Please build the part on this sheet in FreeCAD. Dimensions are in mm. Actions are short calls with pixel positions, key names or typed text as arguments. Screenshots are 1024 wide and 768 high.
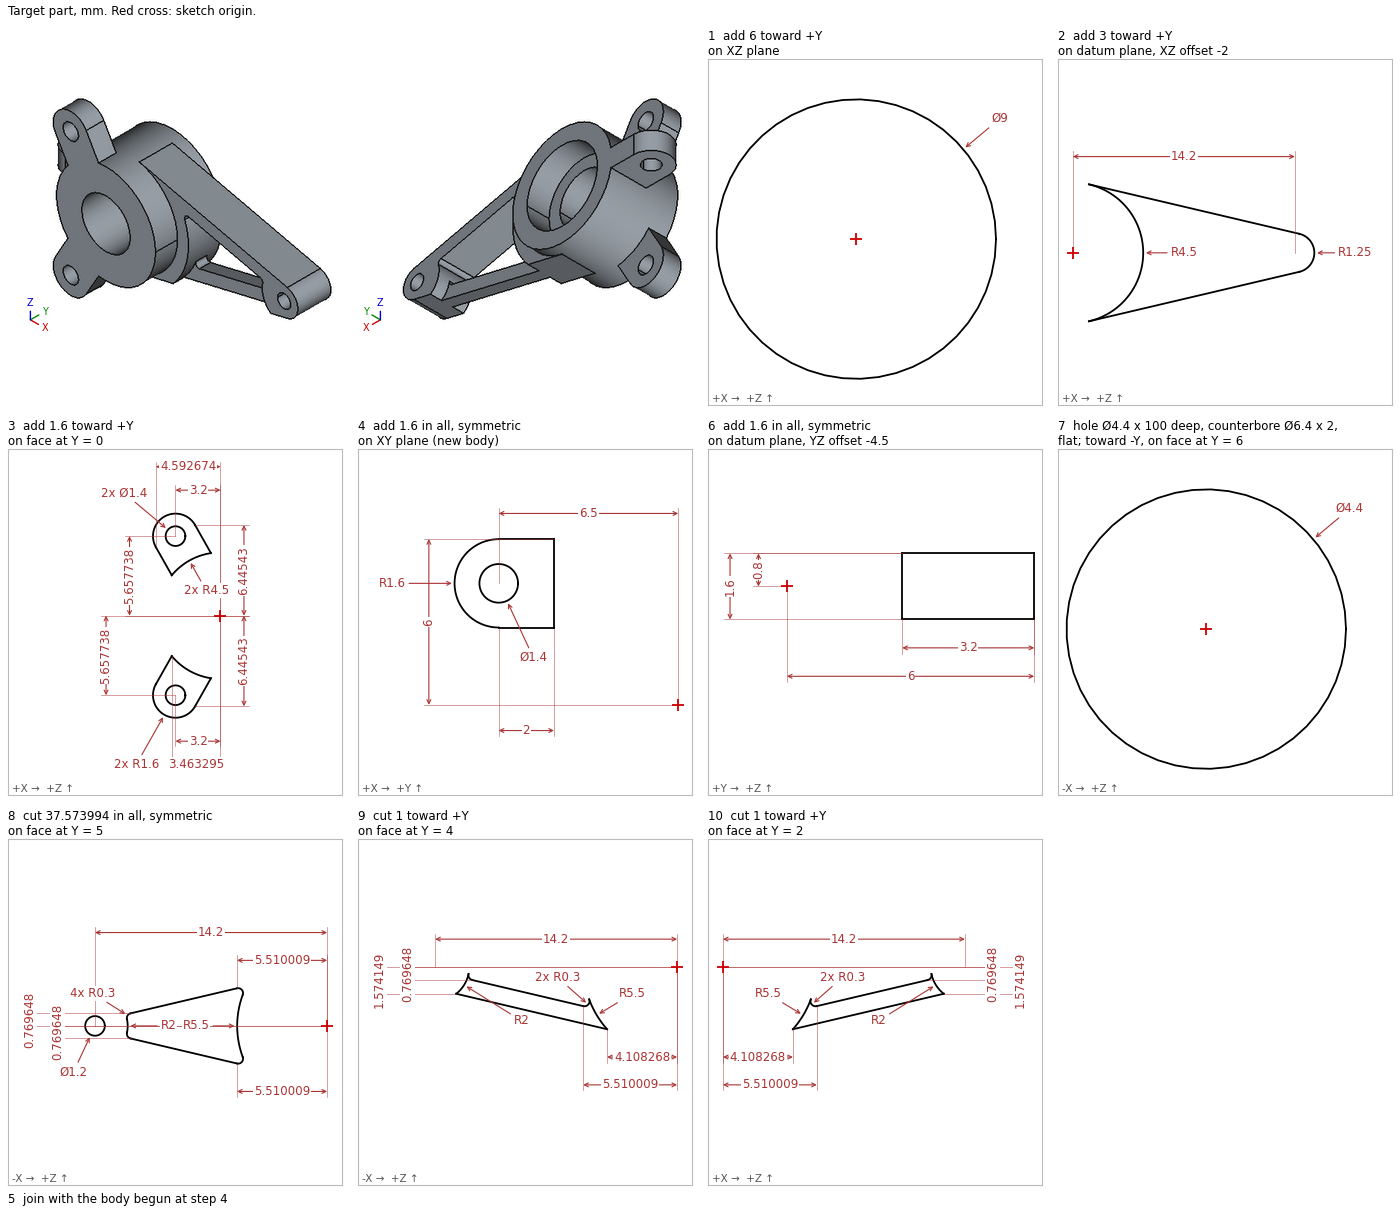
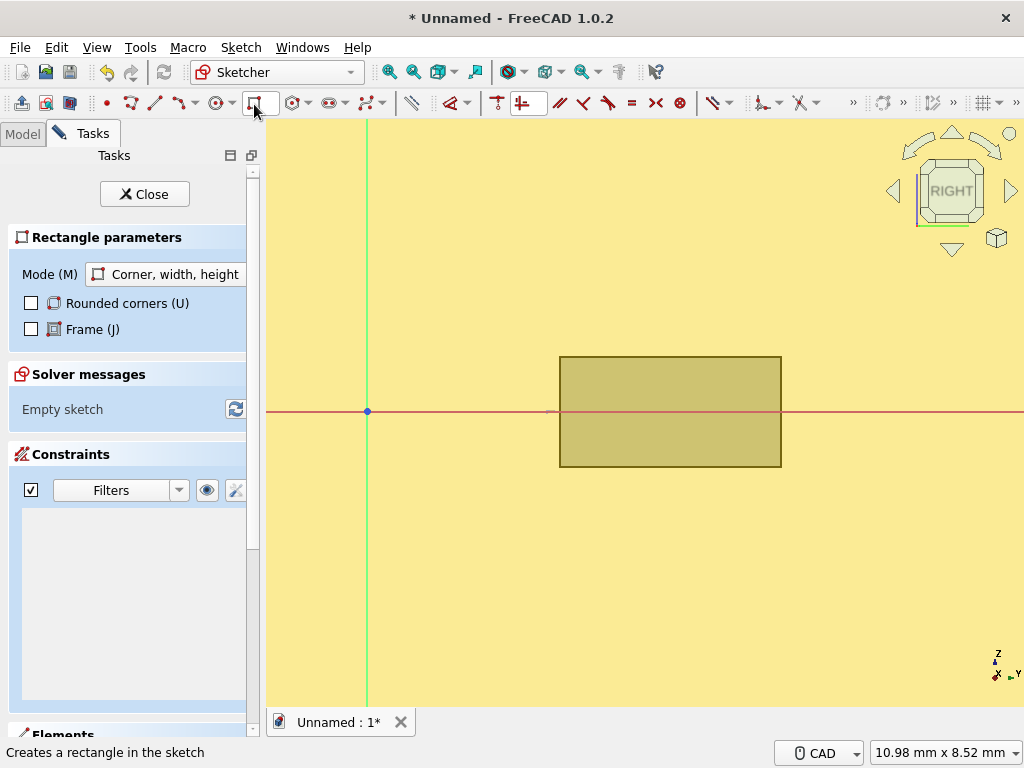
click(560, 357)
click(781, 467)
key(Escape)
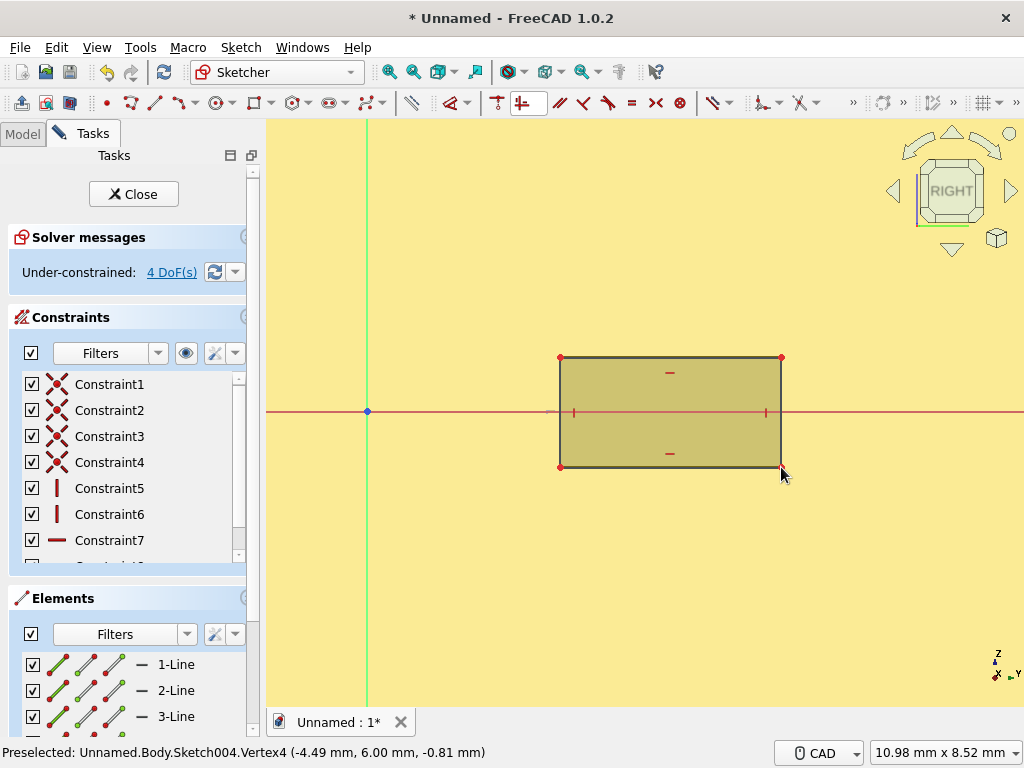
key(d)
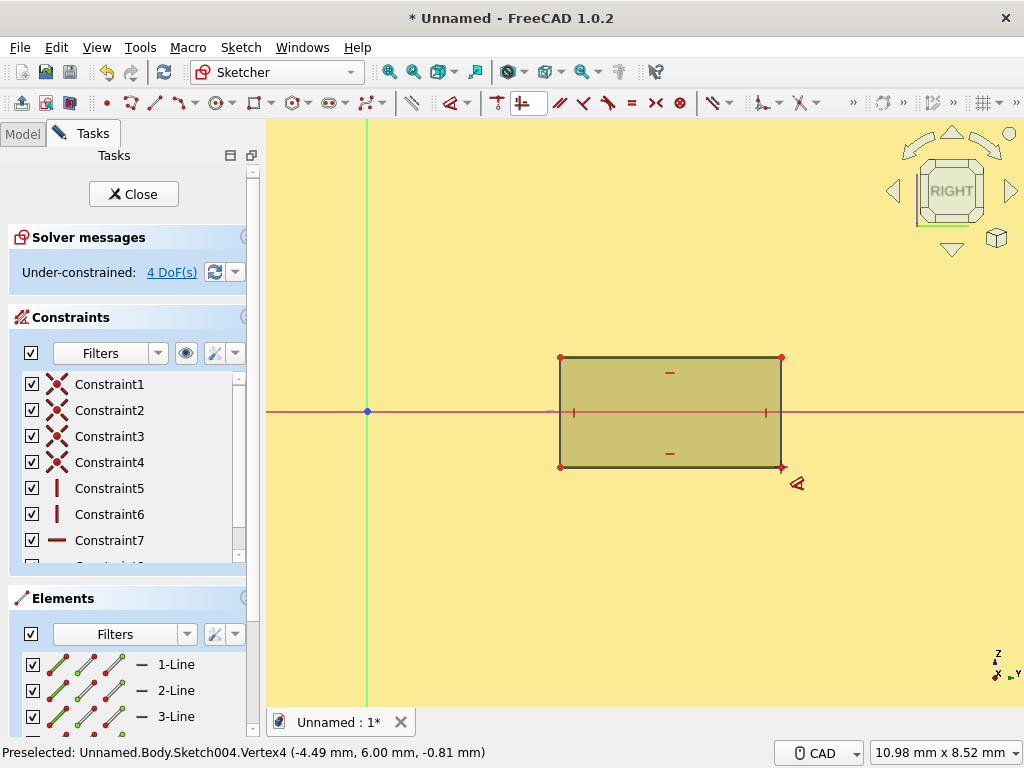
click(781, 468)
click(574, 502)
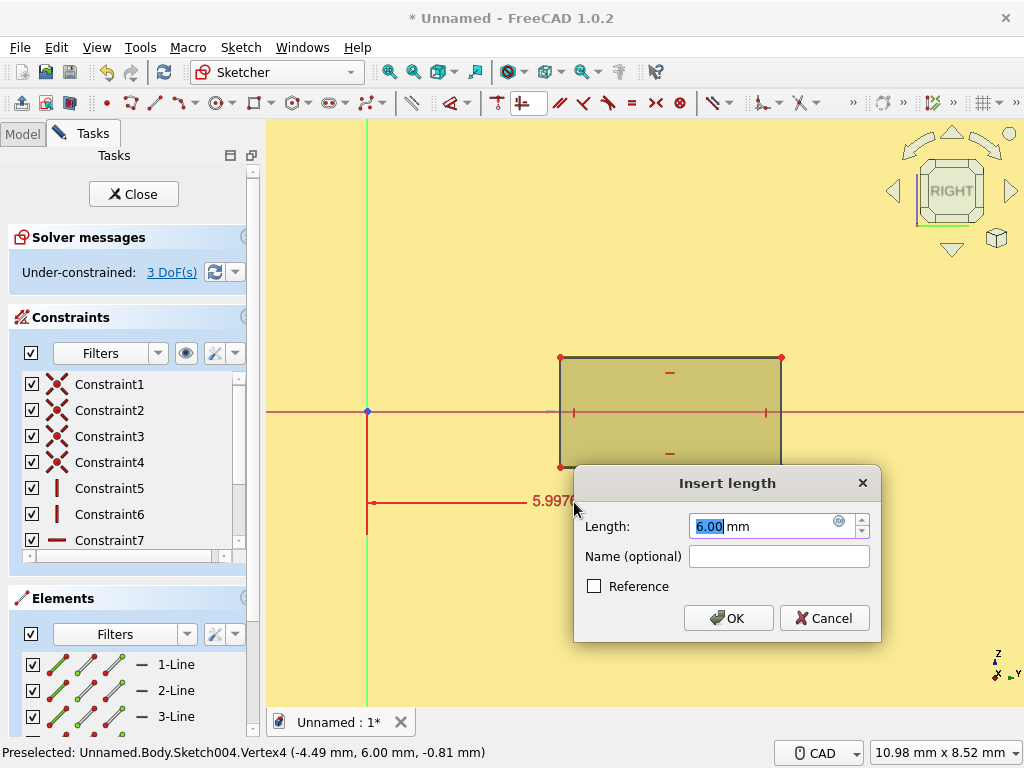
text(6)
key(Return)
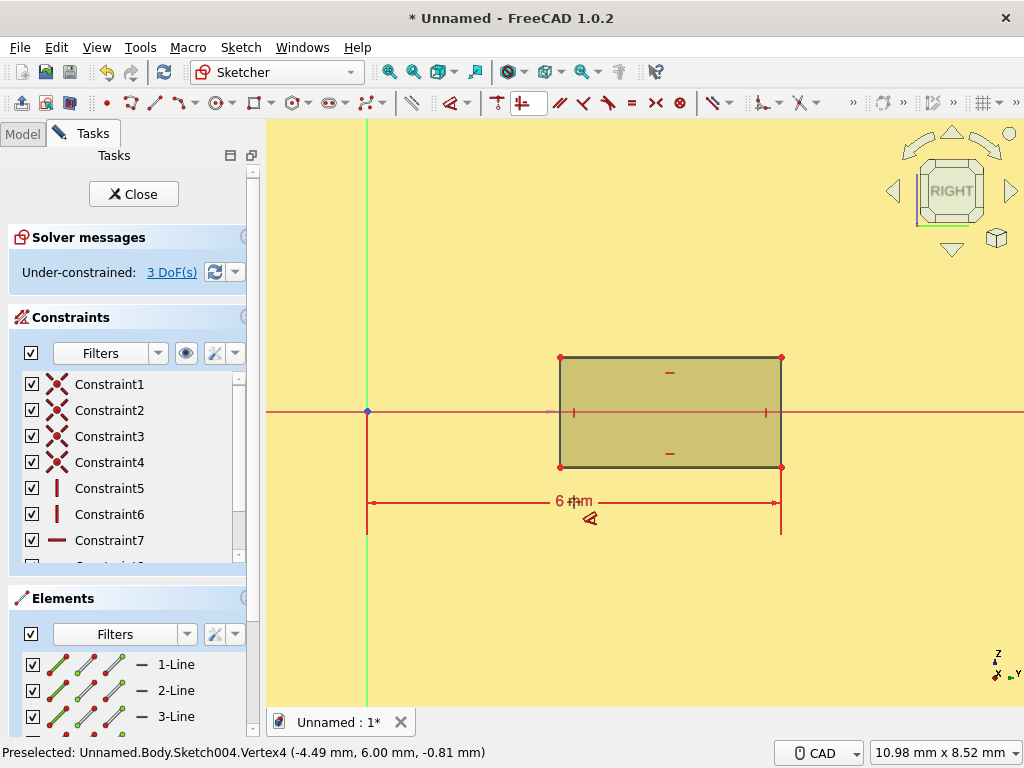
click(560, 391)
click(526, 388)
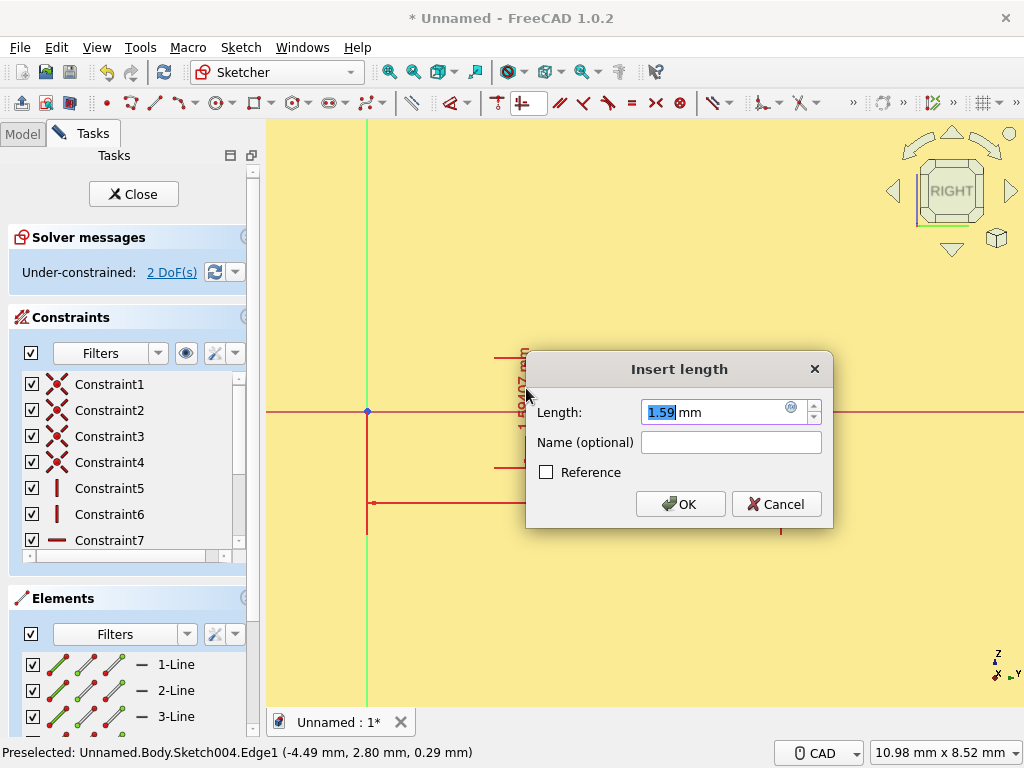
text(1.6)
key(Return)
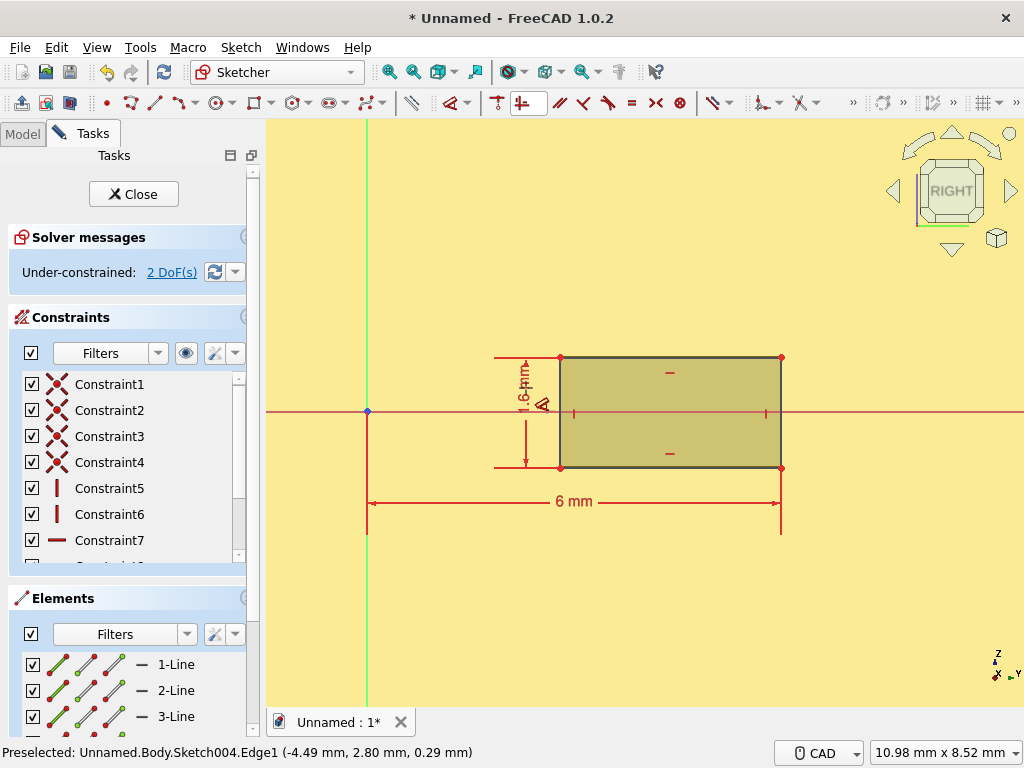
click(626, 468)
click(671, 502)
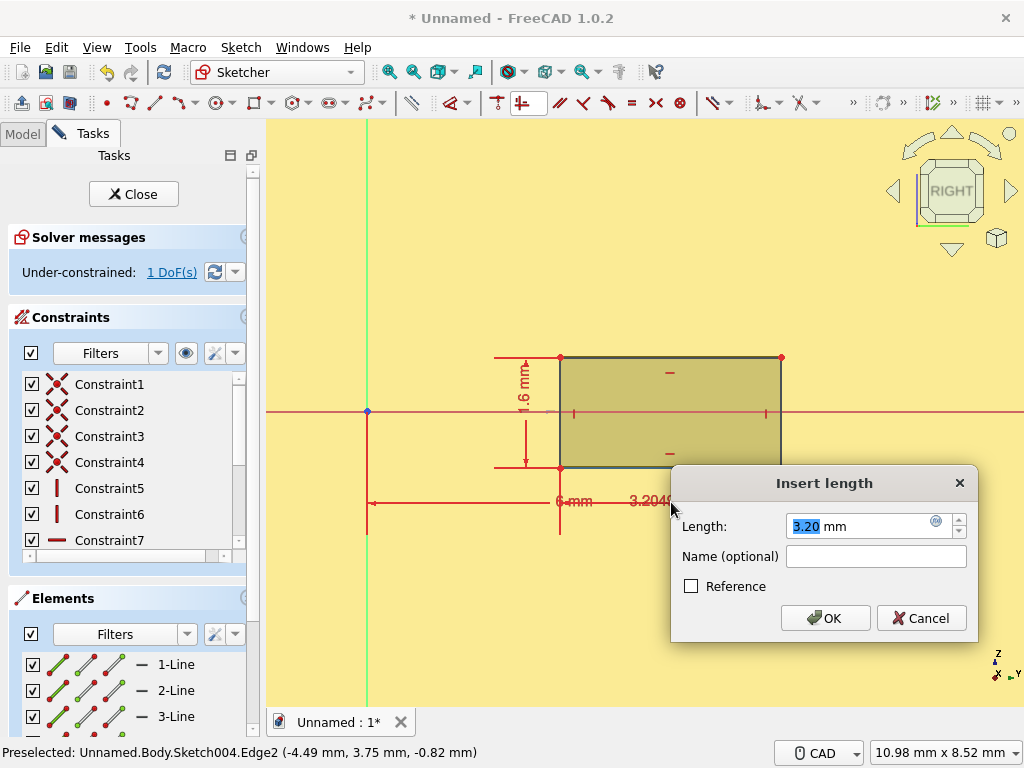
text(3.2)
key(Return)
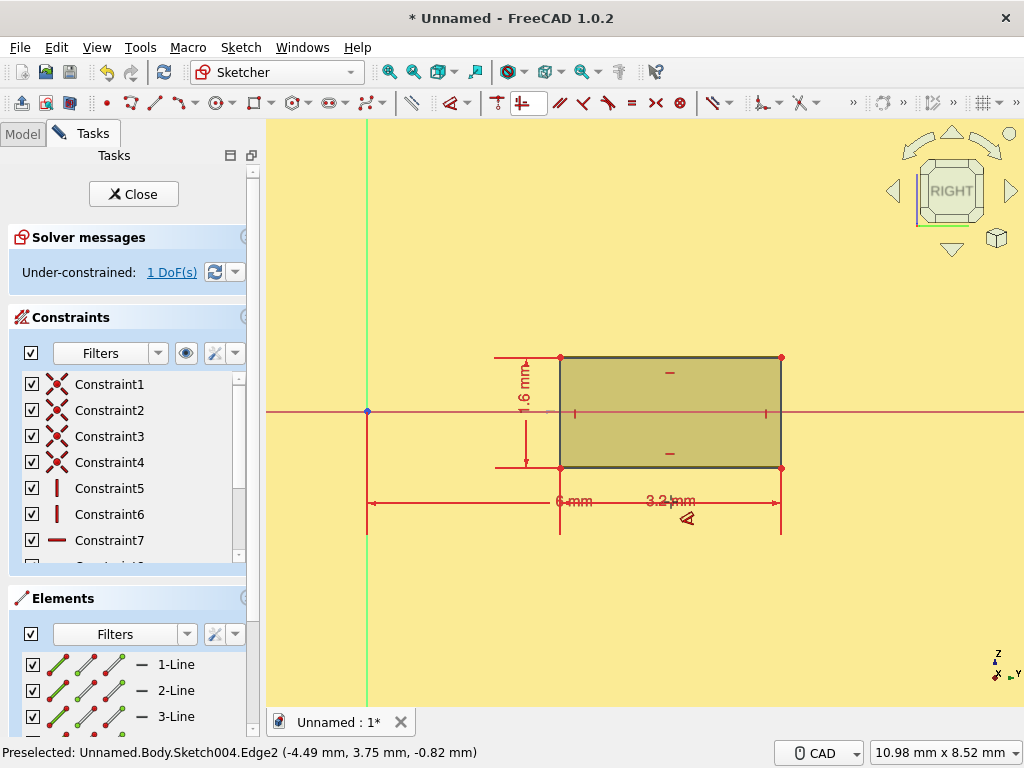
click(560, 358)
click(333, 385)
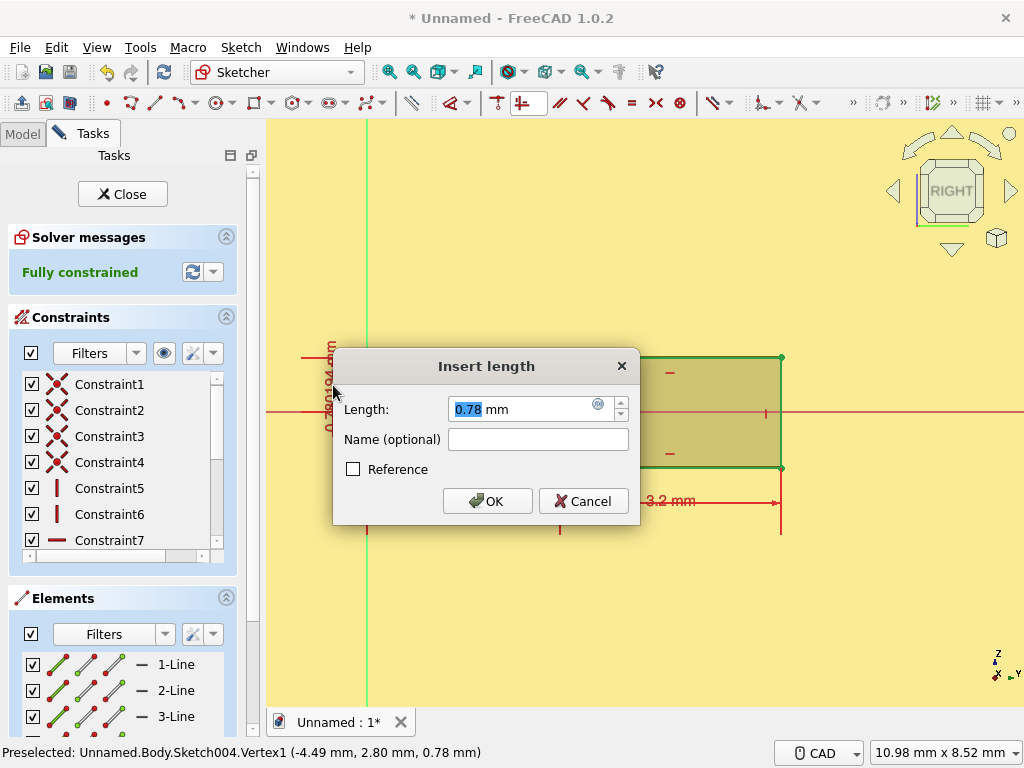
text(0.8)
key(Return)
key(Escape)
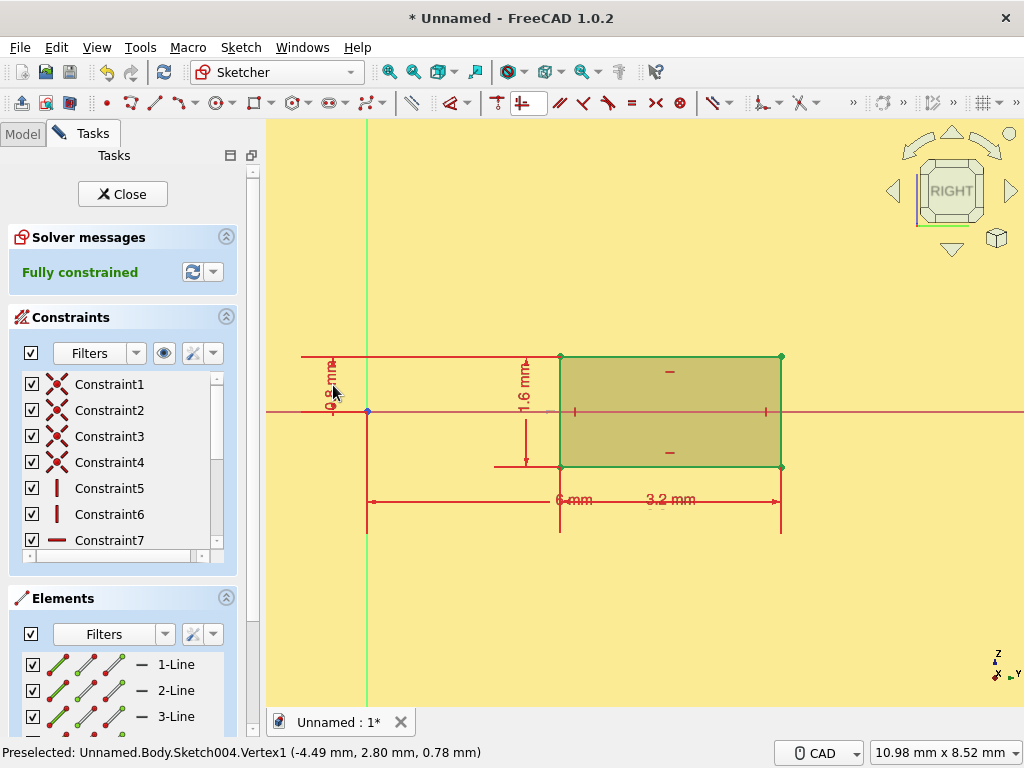
click(123, 194)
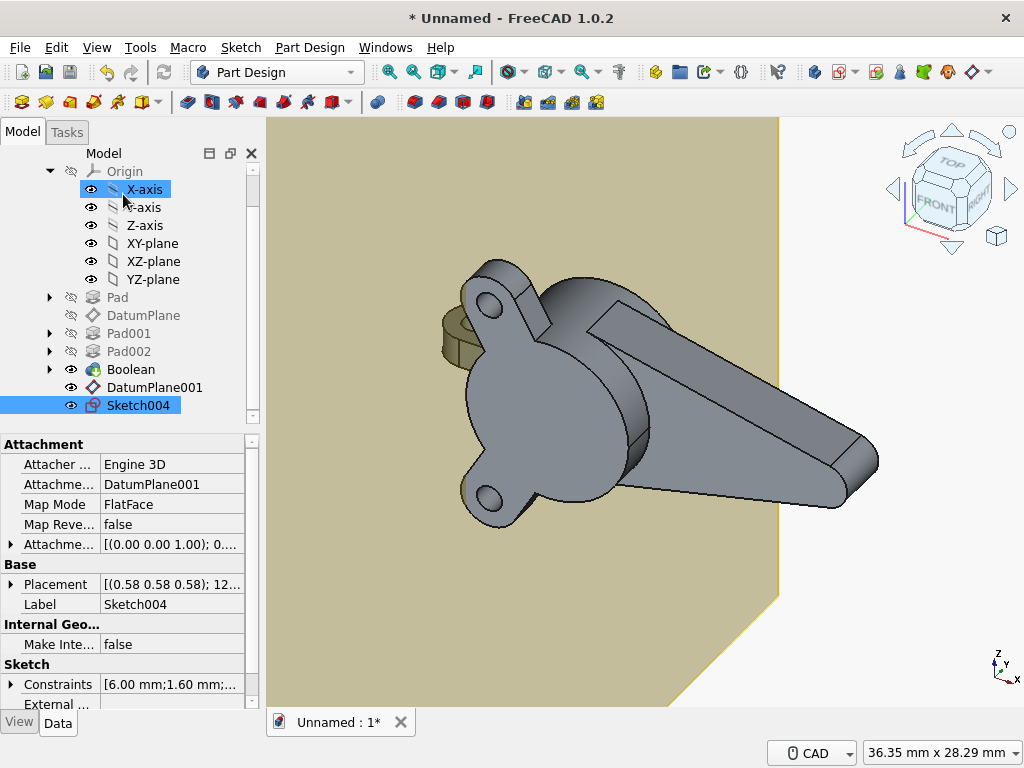
click(22, 102)